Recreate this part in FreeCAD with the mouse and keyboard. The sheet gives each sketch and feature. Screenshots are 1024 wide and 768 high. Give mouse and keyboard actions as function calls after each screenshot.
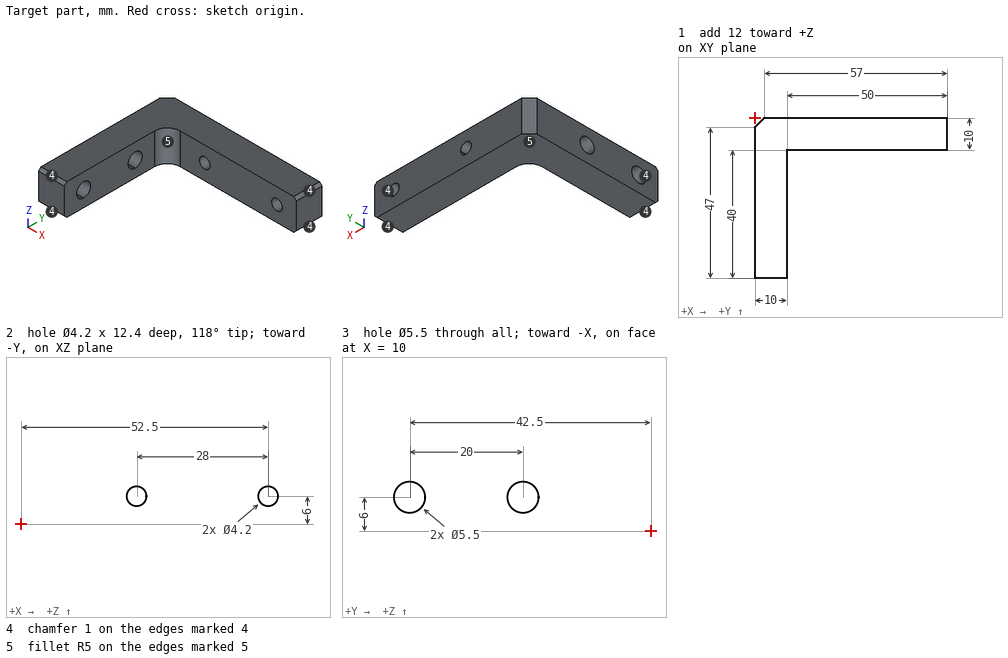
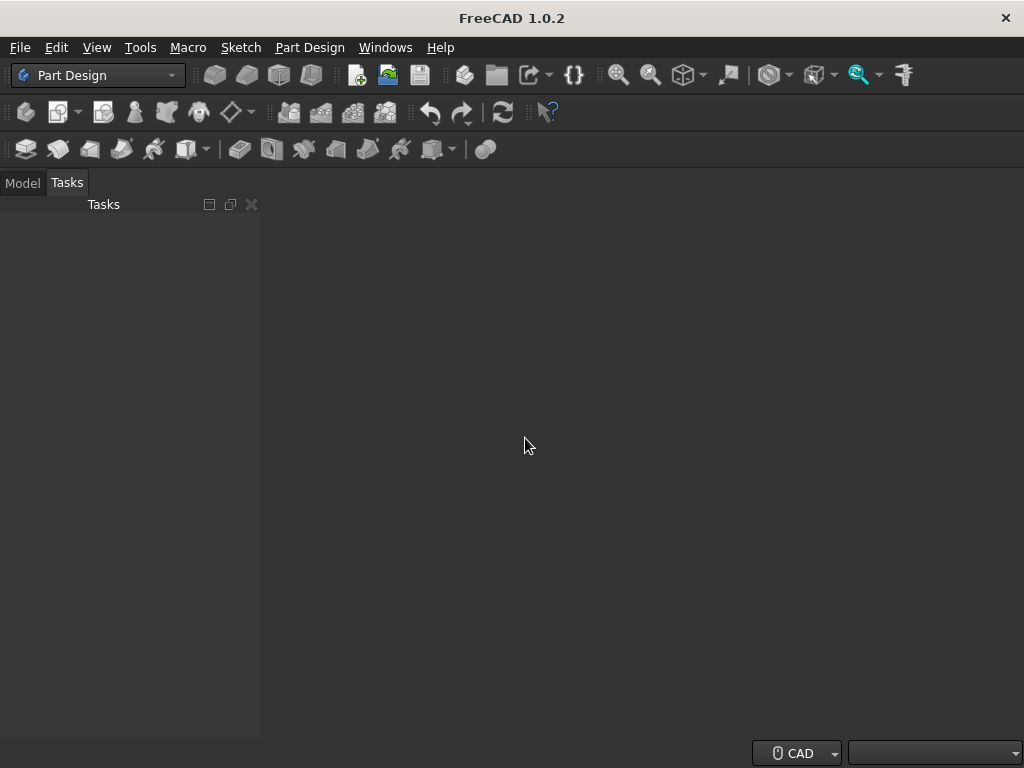
key(ctrl+n)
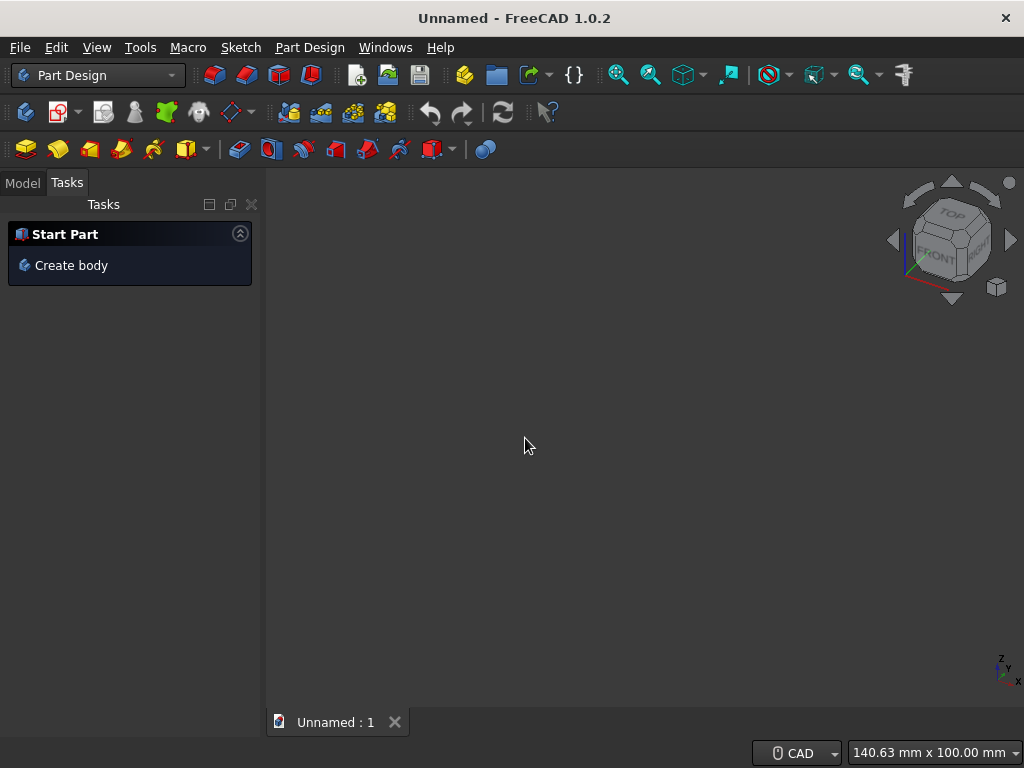
click(58, 112)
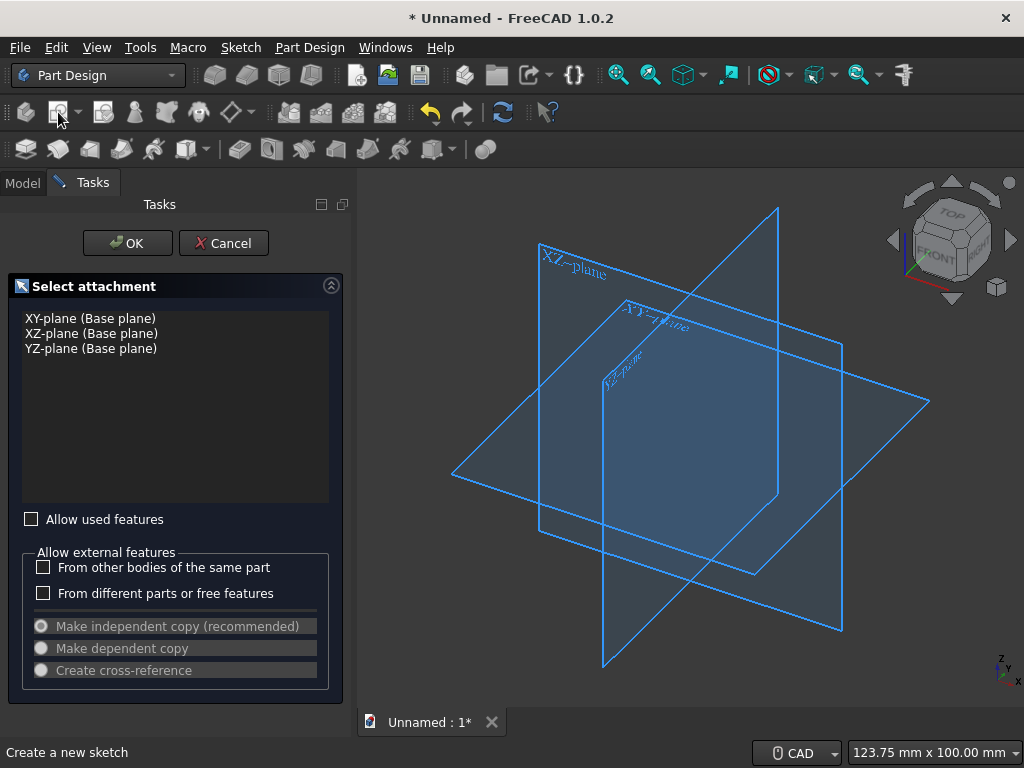
click(82, 318)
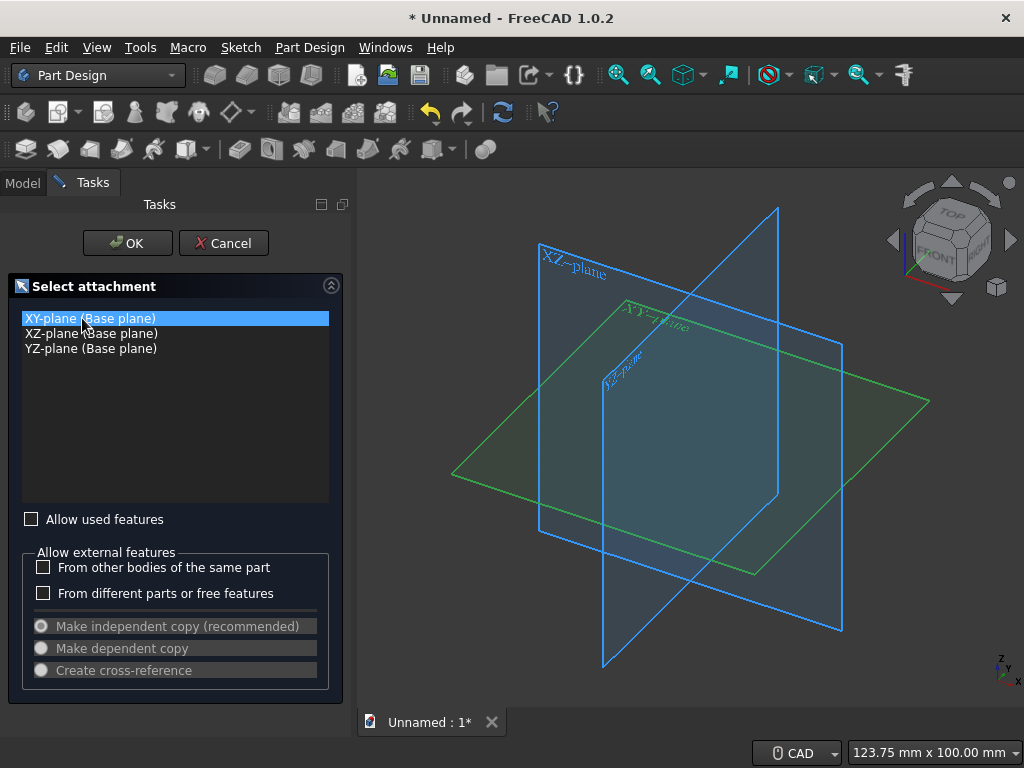
click(128, 243)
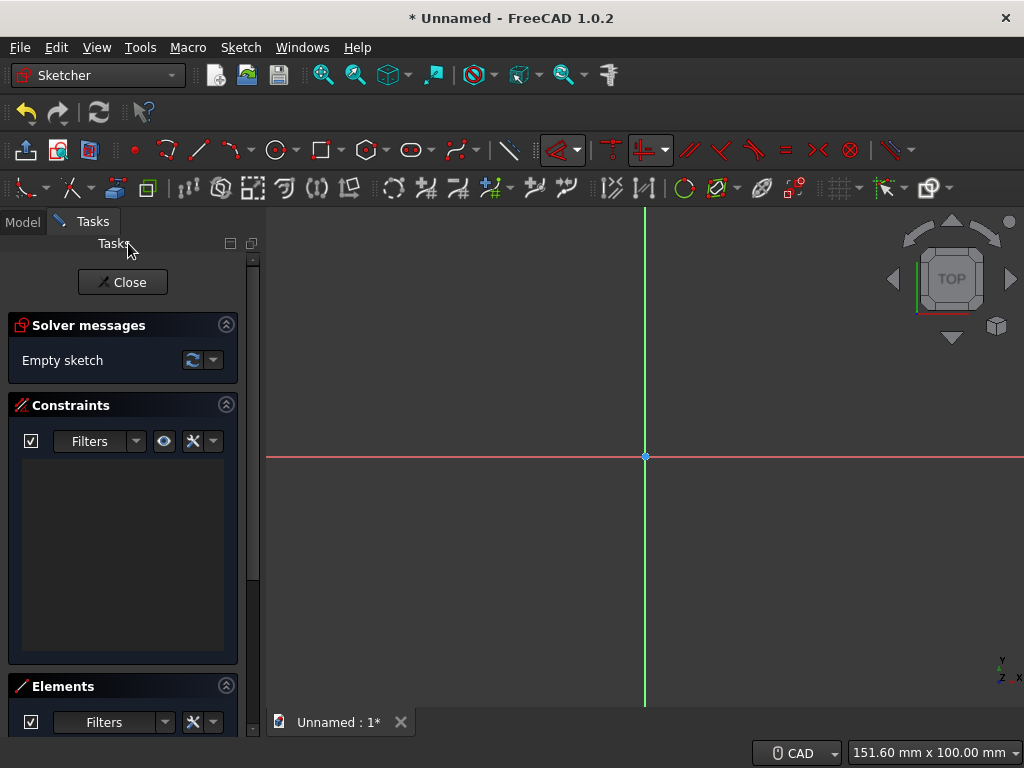
scroll(294, 235, down, 1)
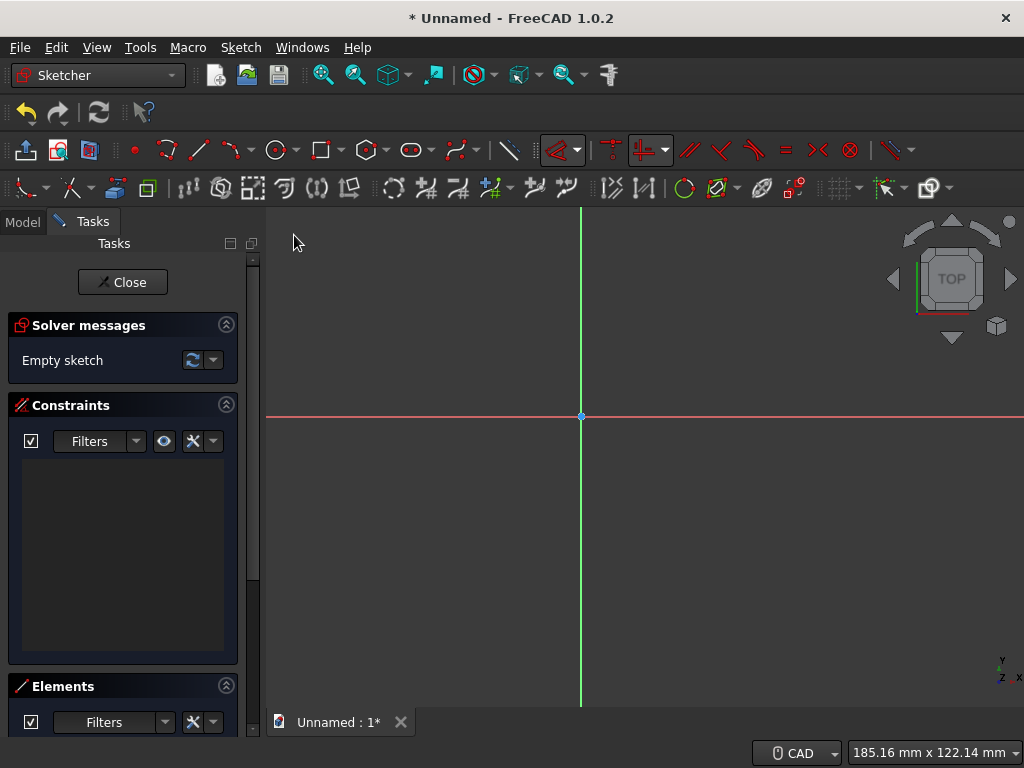
scroll(859, 645, up, 2)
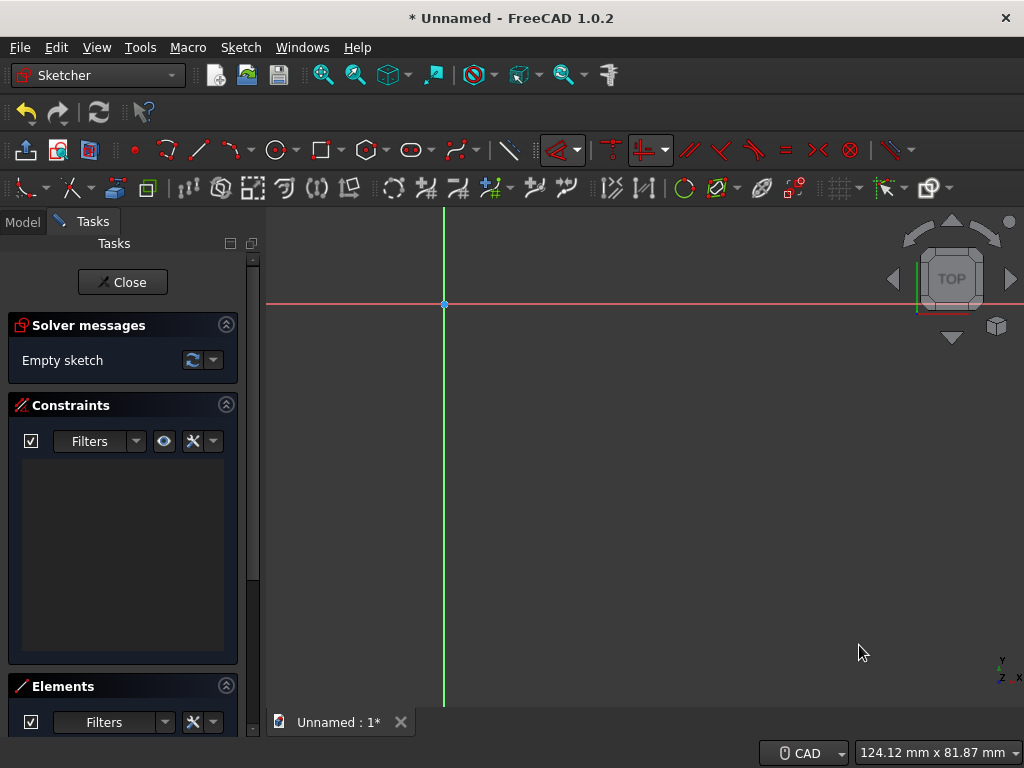
click(168, 150)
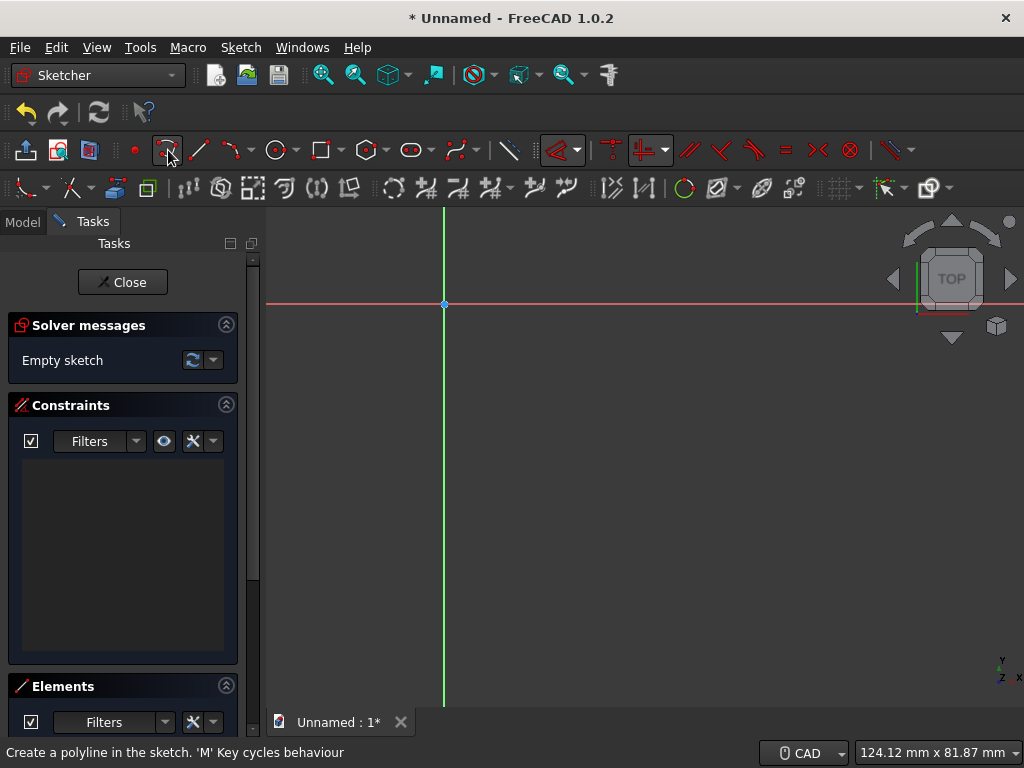
click(463, 304)
click(444, 322)
click(453, 609)
click(506, 609)
click(506, 365)
click(811, 365)
click(811, 313)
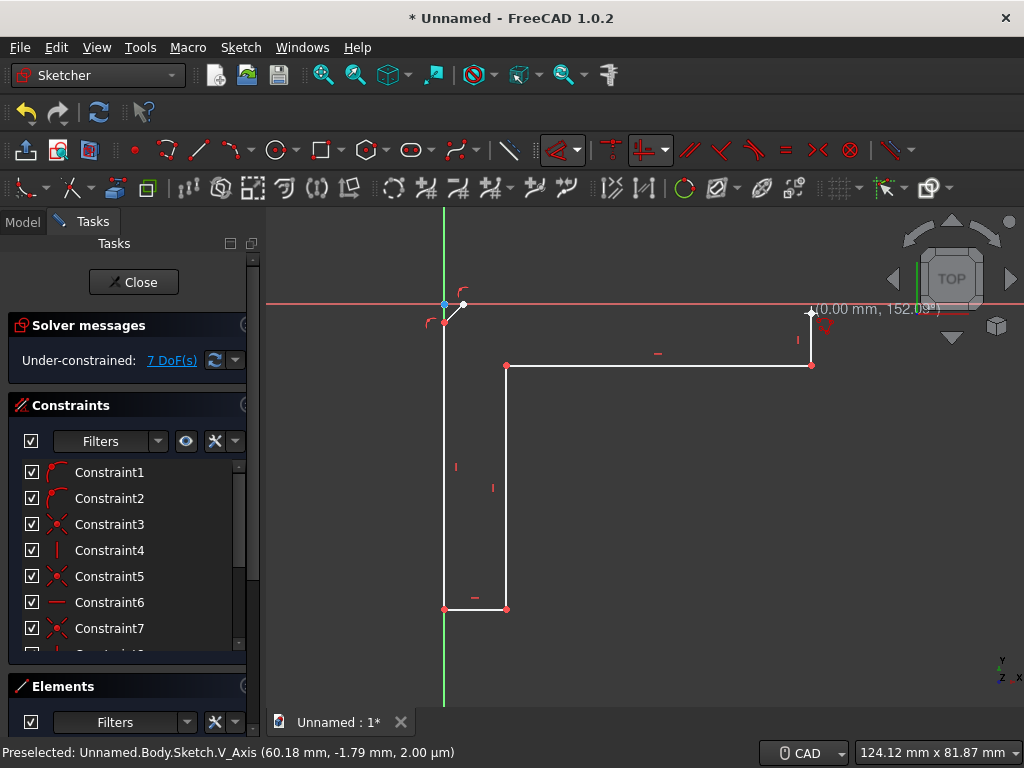
scroll(463, 304, up, 2)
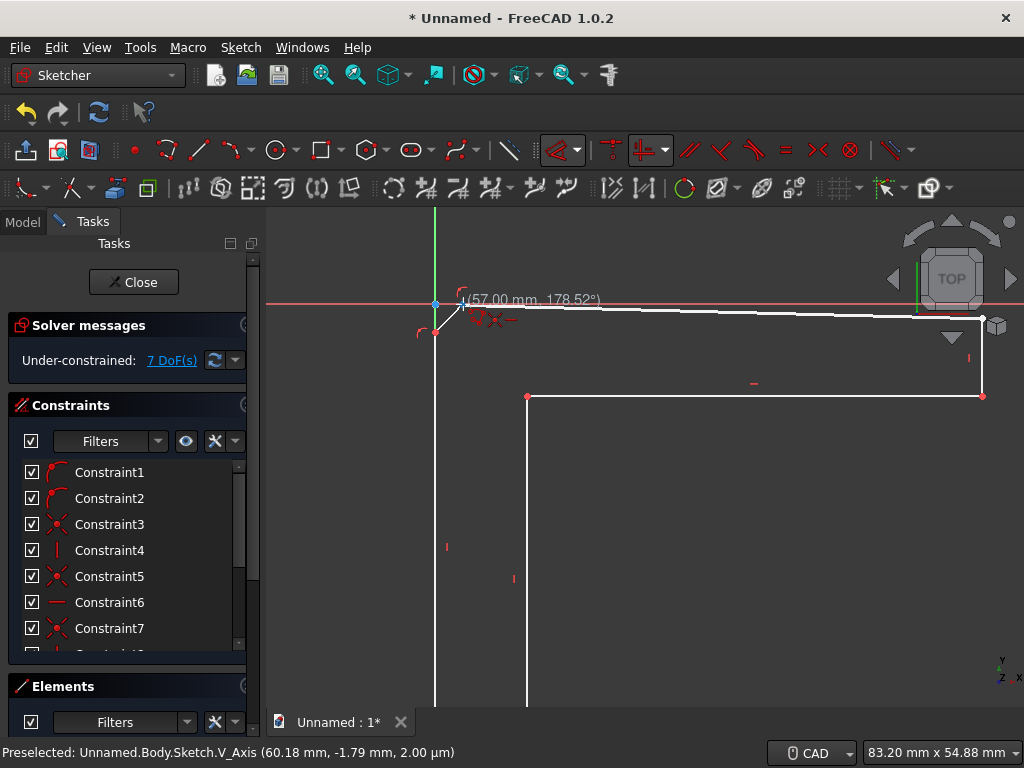
click(463, 304)
key(Escape)
key(Escape)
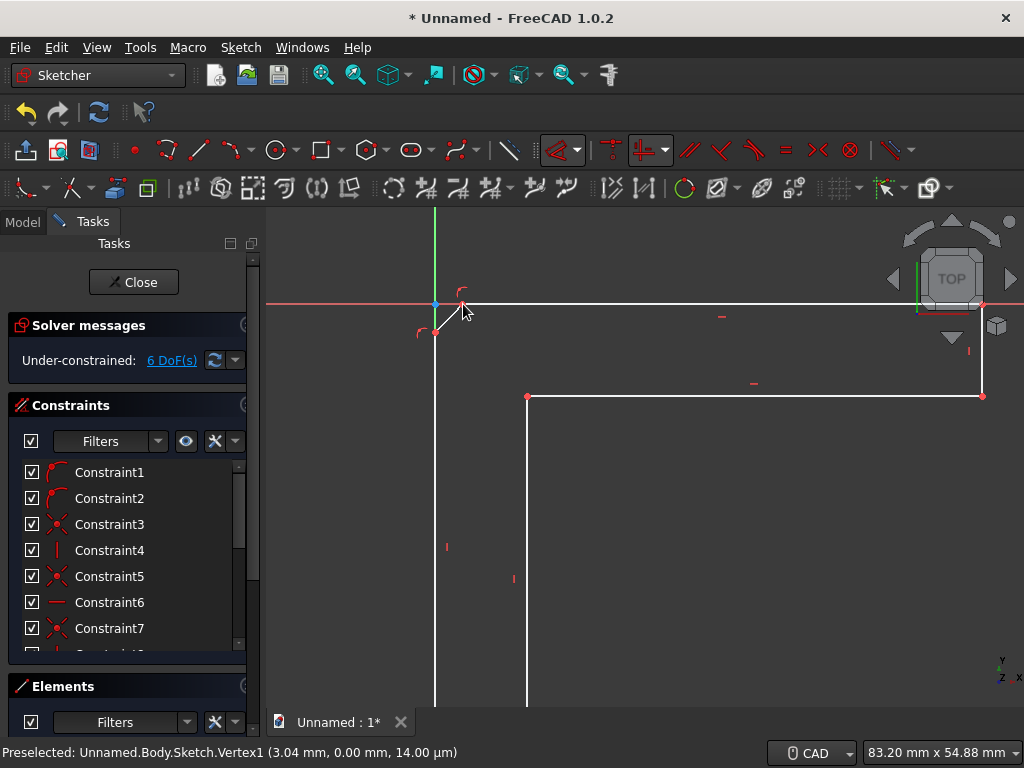
key(d)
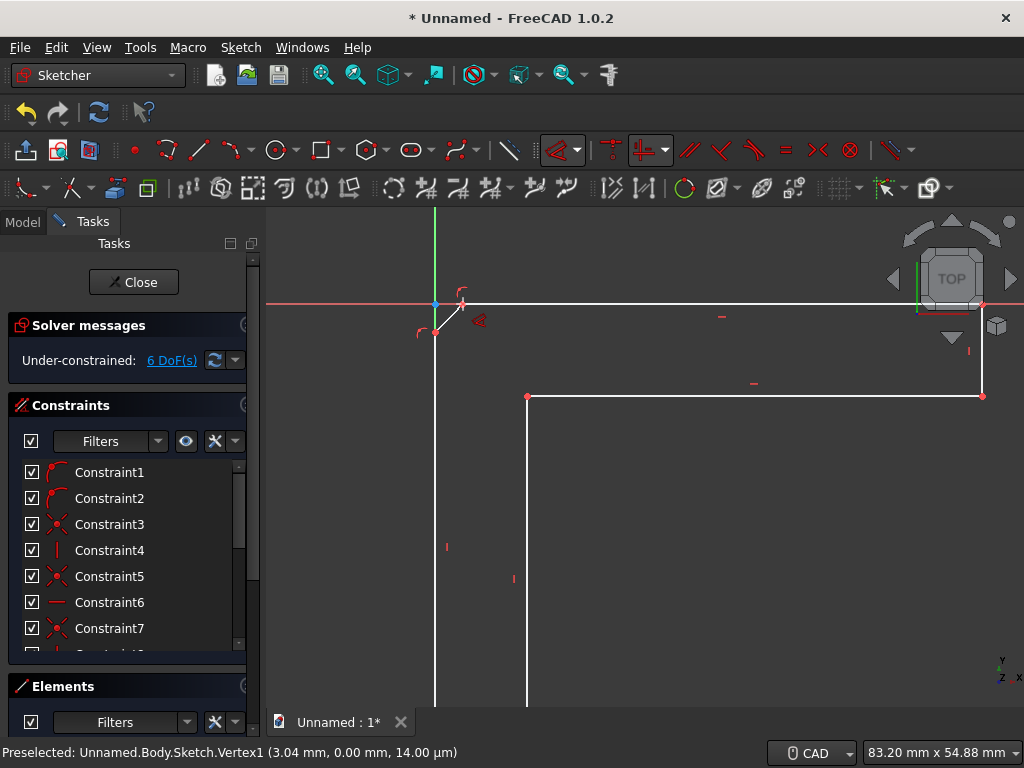
click(435, 461)
click(401, 506)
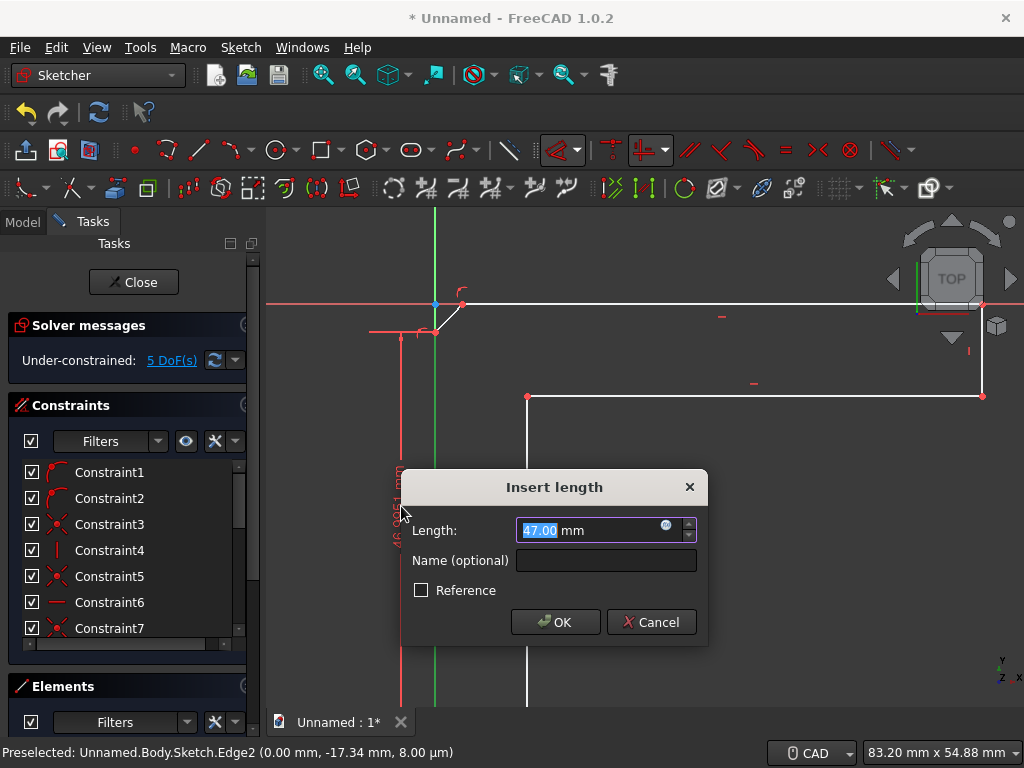
text(47)
key(Return)